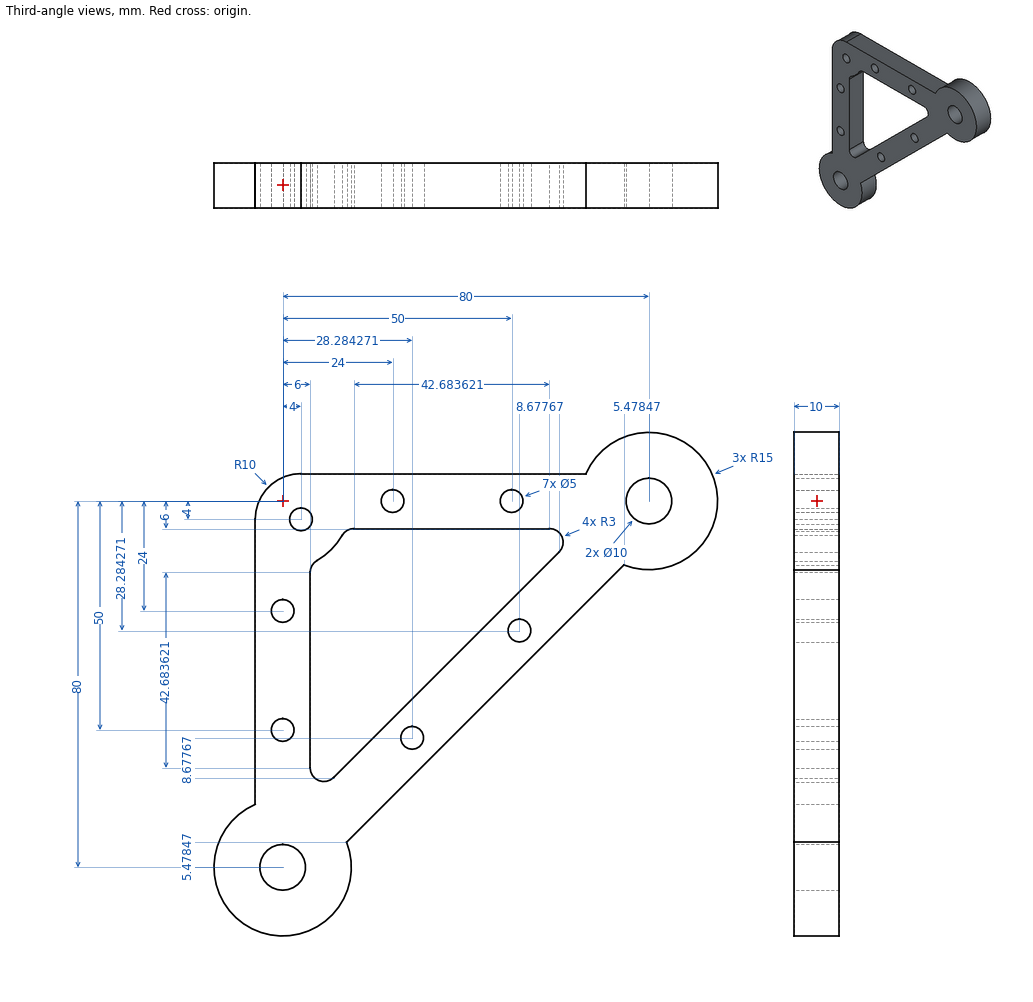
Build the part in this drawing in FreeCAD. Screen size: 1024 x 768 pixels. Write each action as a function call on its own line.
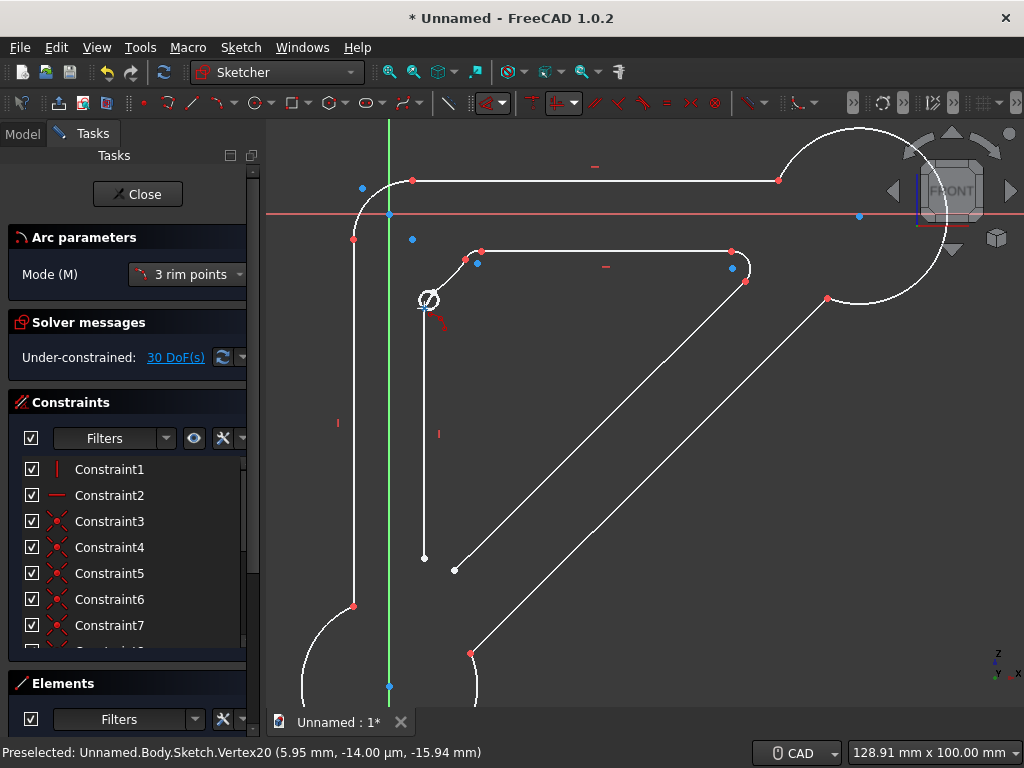
scroll(427, 297, up, 10)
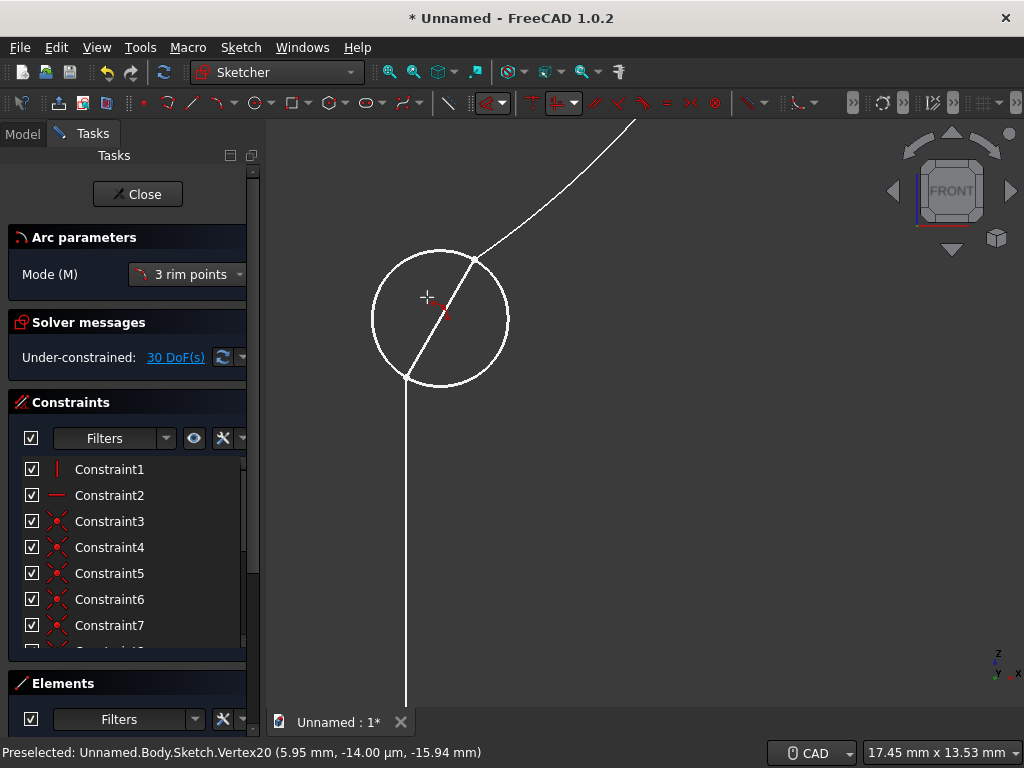
click(426, 297)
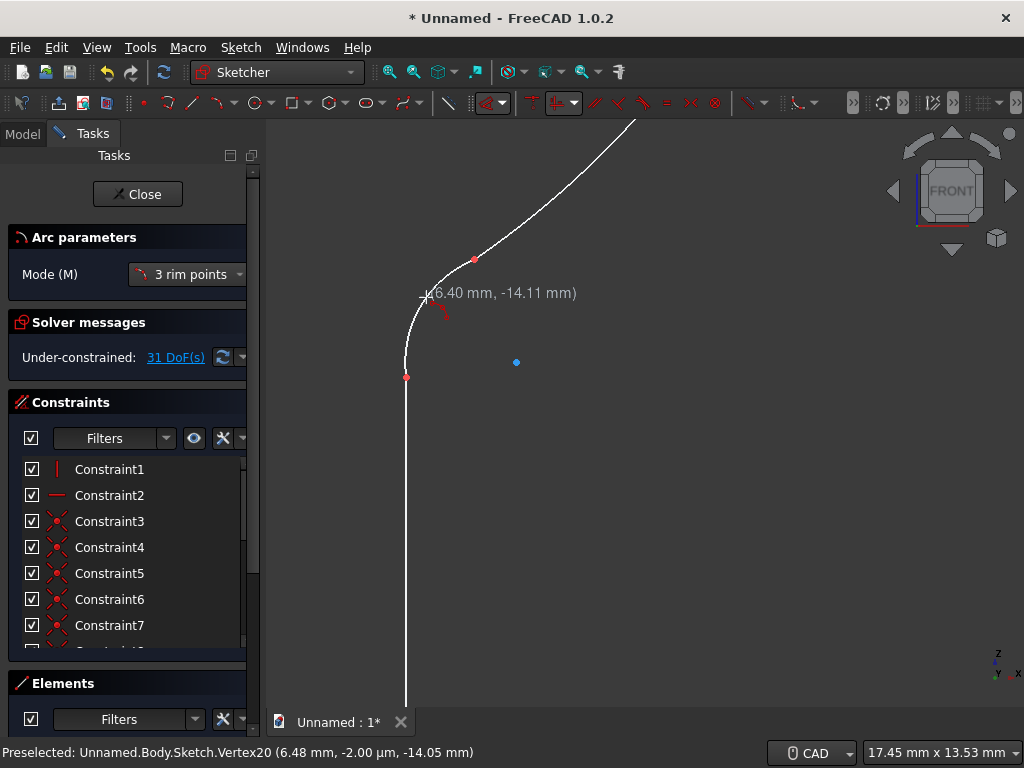
scroll(429, 295, down, 12)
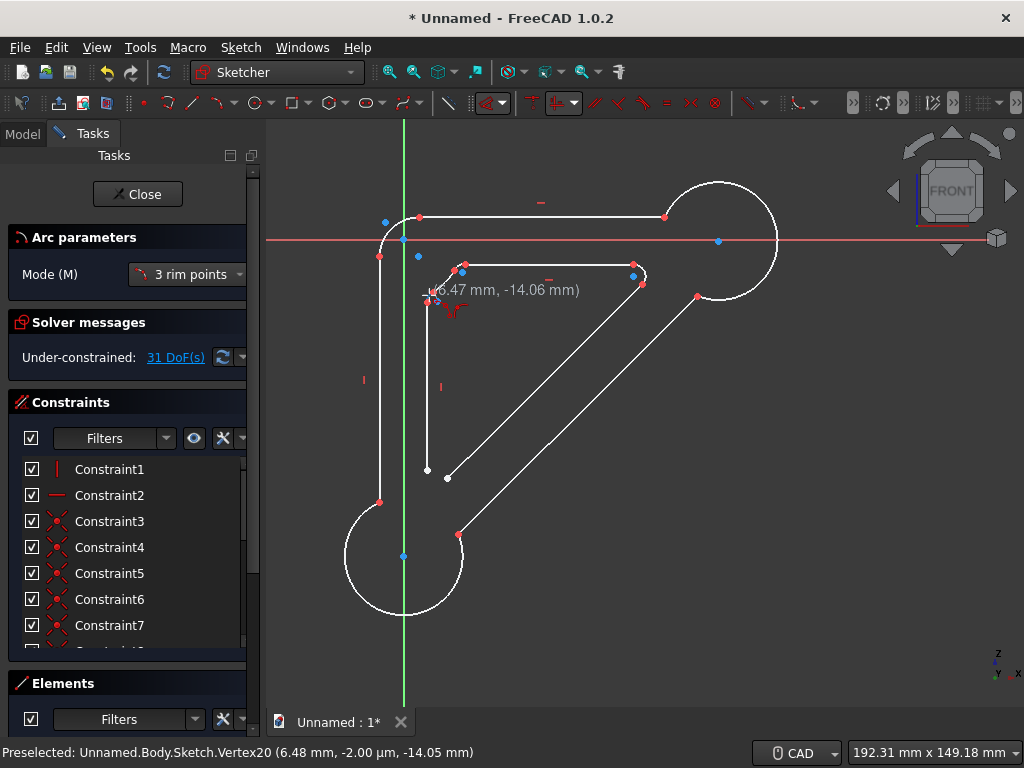
click(427, 471)
click(447, 479)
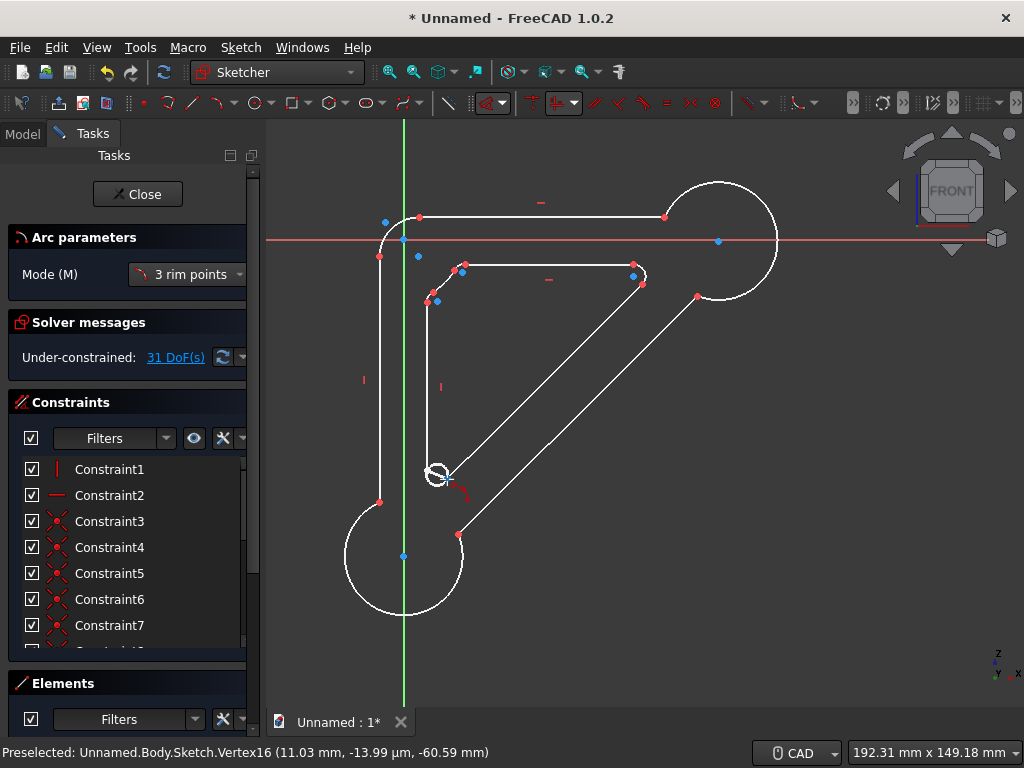
scroll(435, 481, up, 4)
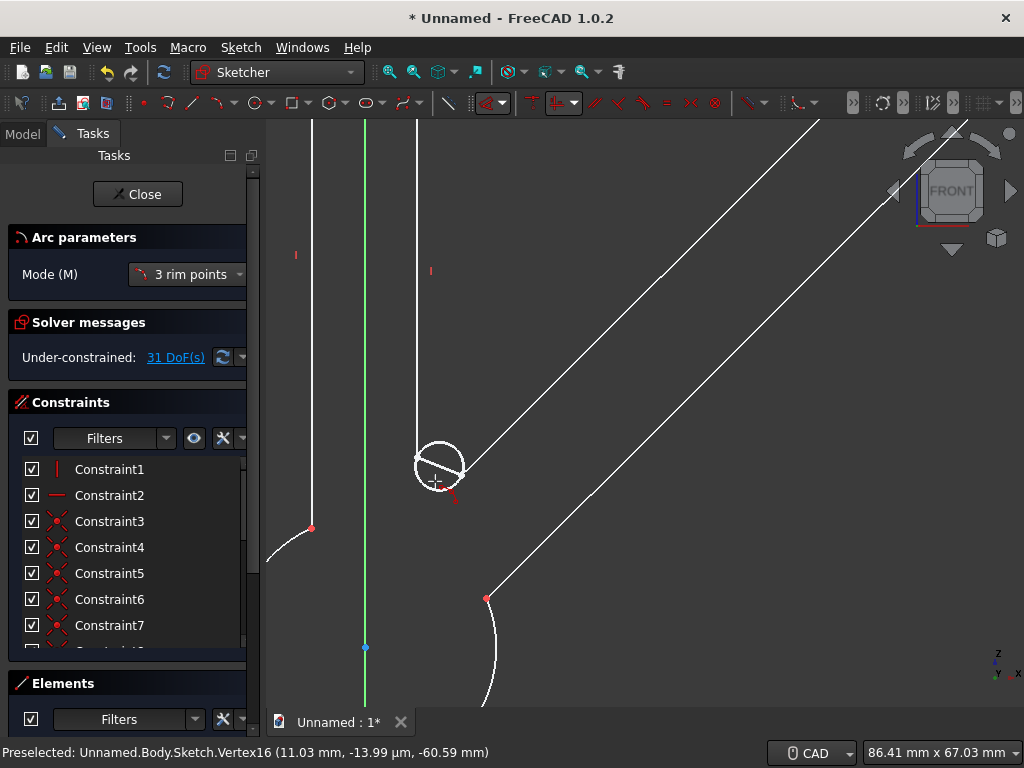
click(434, 479)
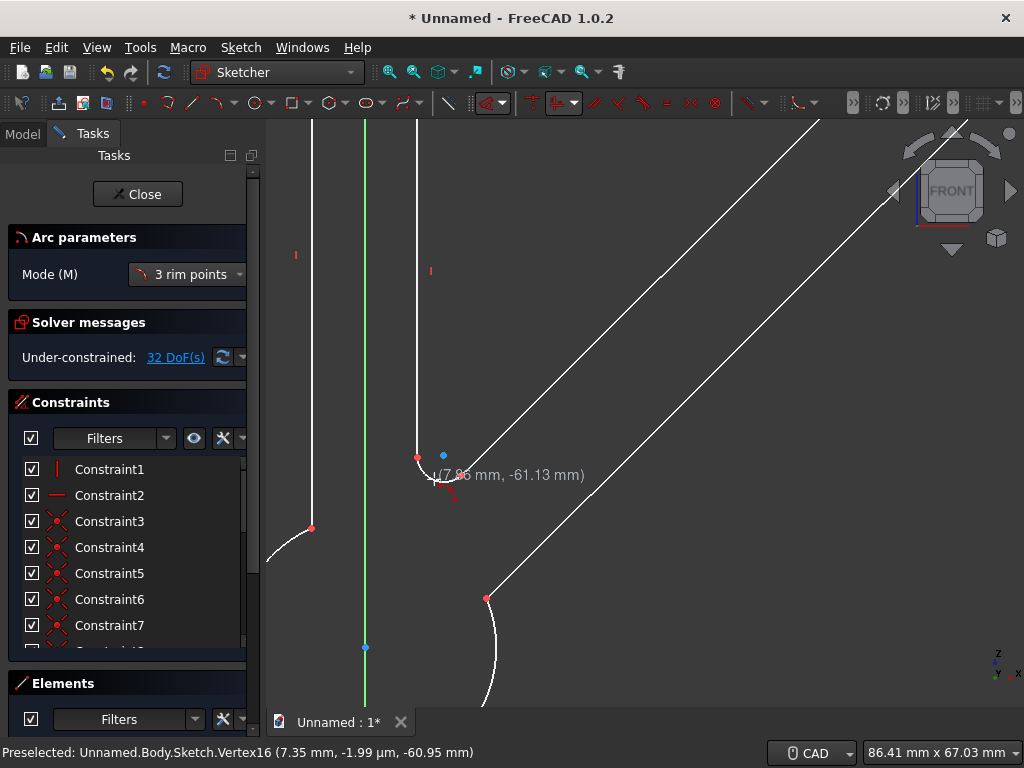
click(256, 104)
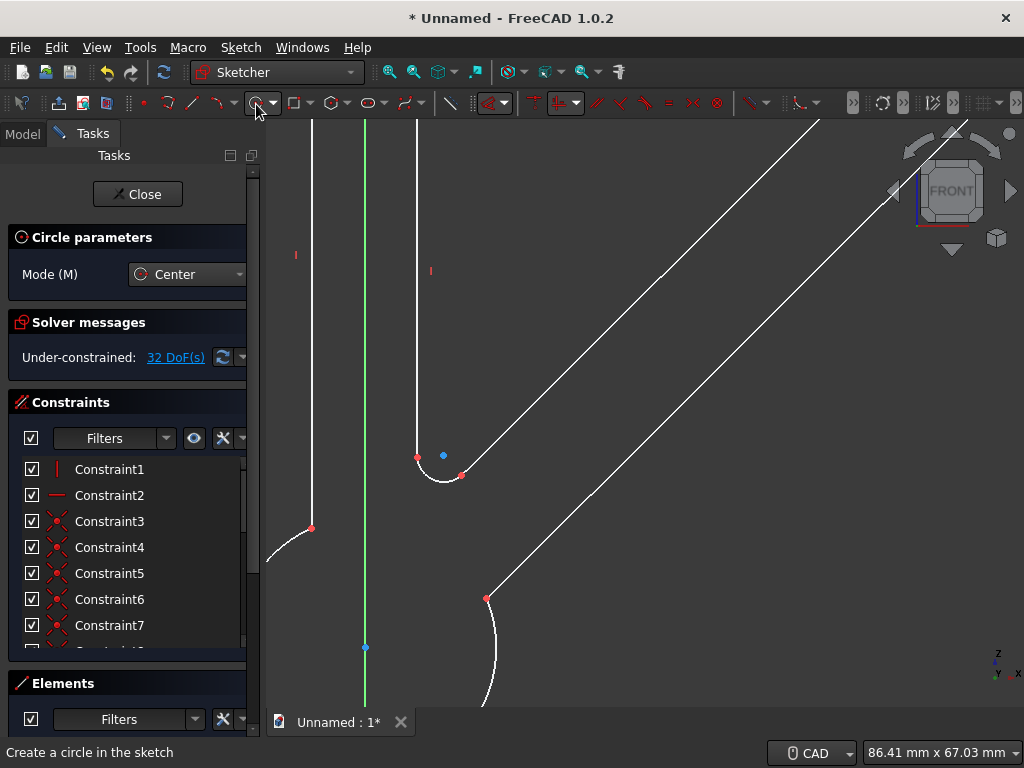
scroll(435, 481, down, 4)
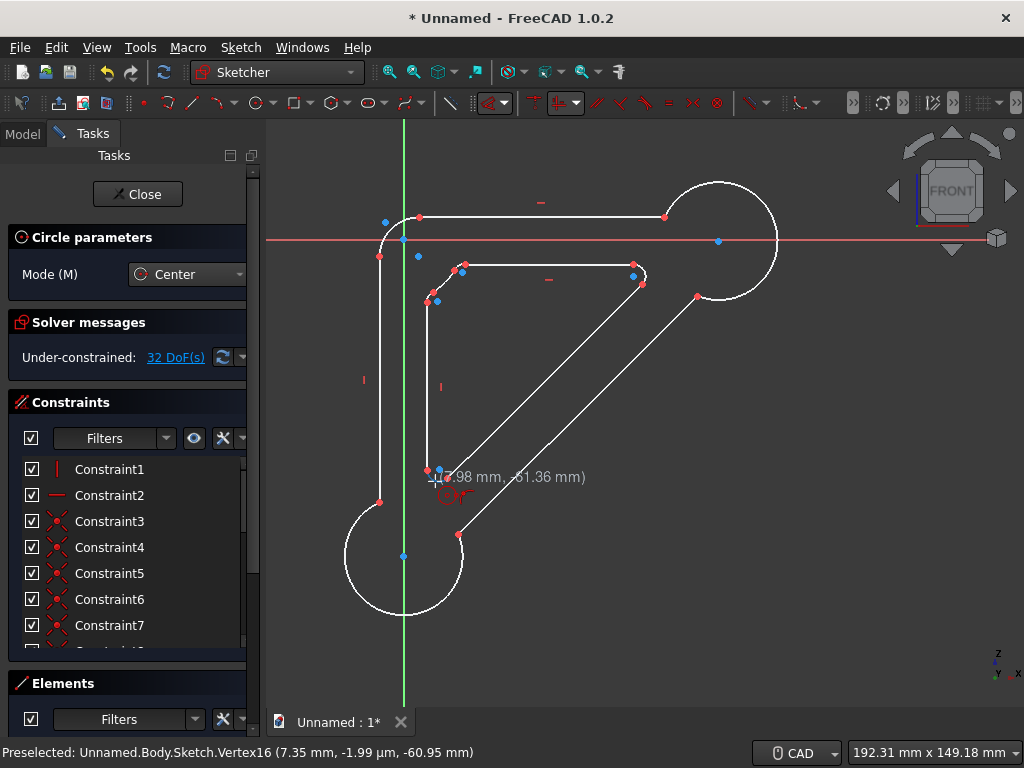
click(719, 240)
click(726, 221)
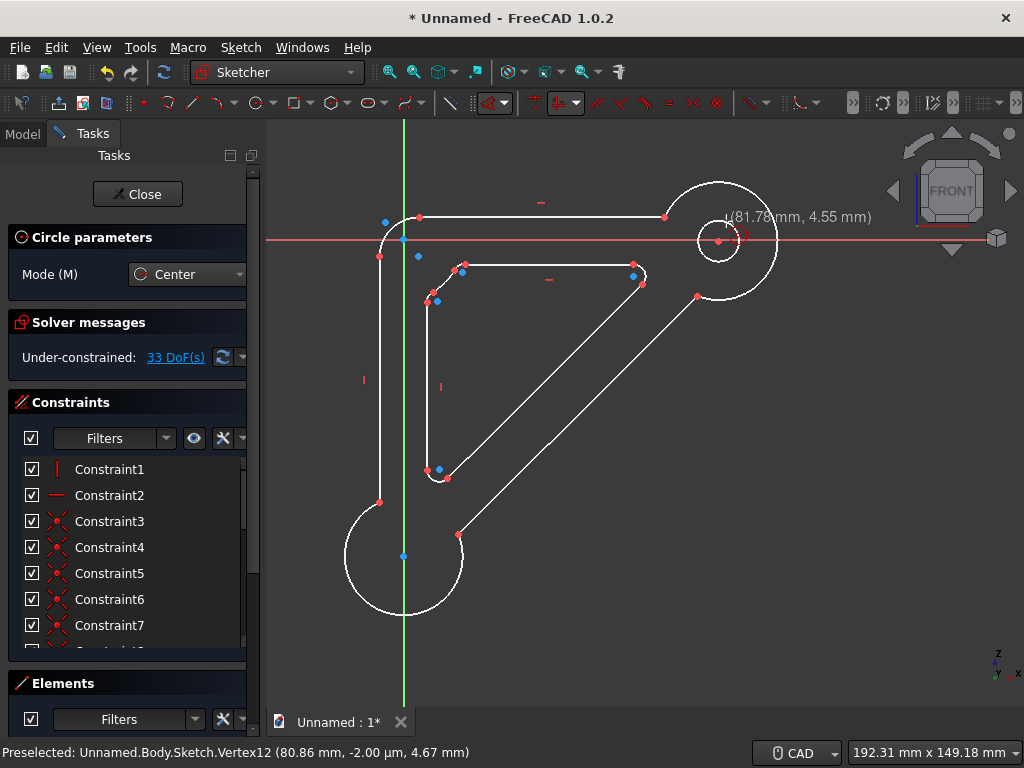
scroll(601, 240, up, 5)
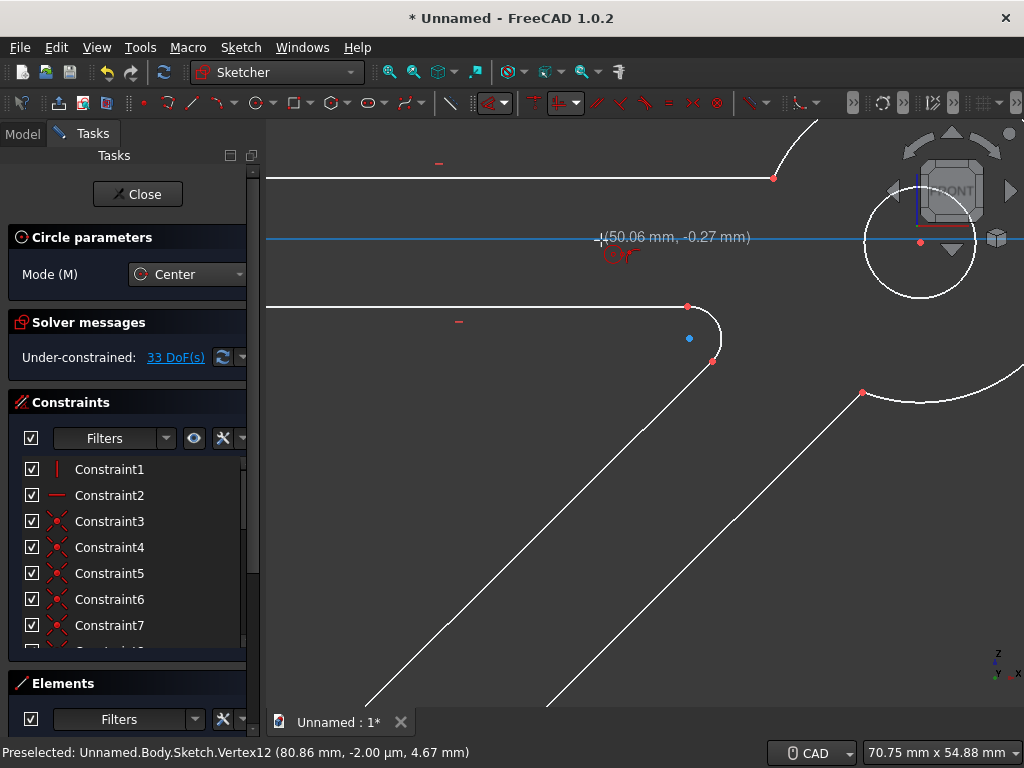
click(600, 239)
click(619, 221)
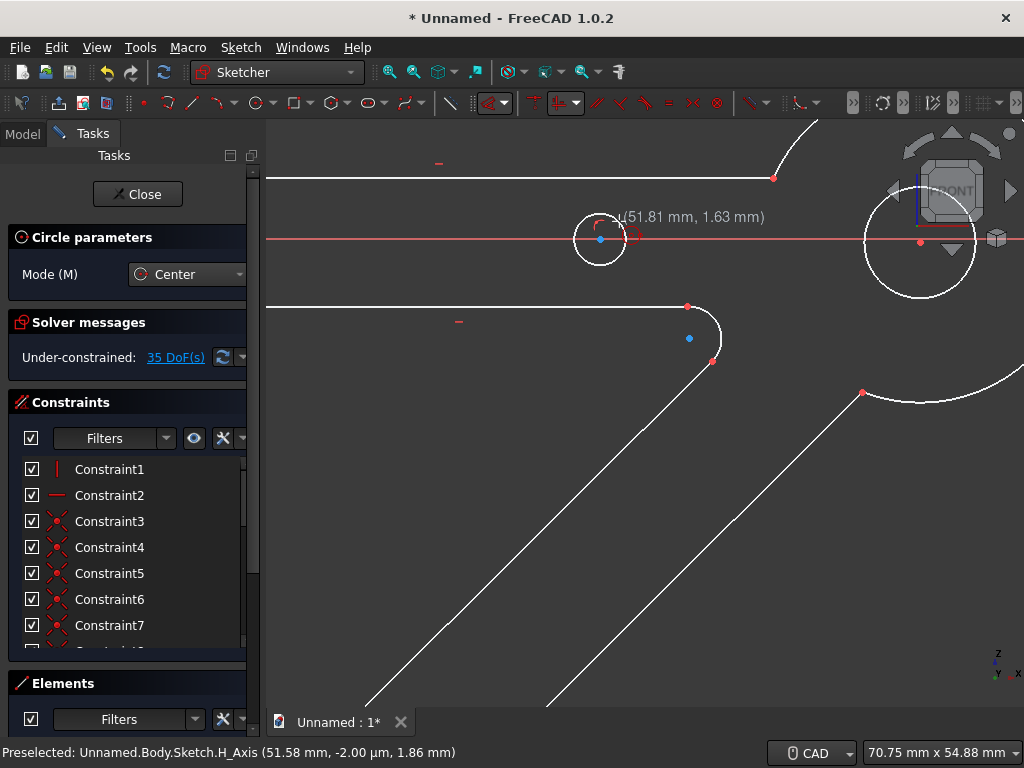
click(618, 543)
click(637, 524)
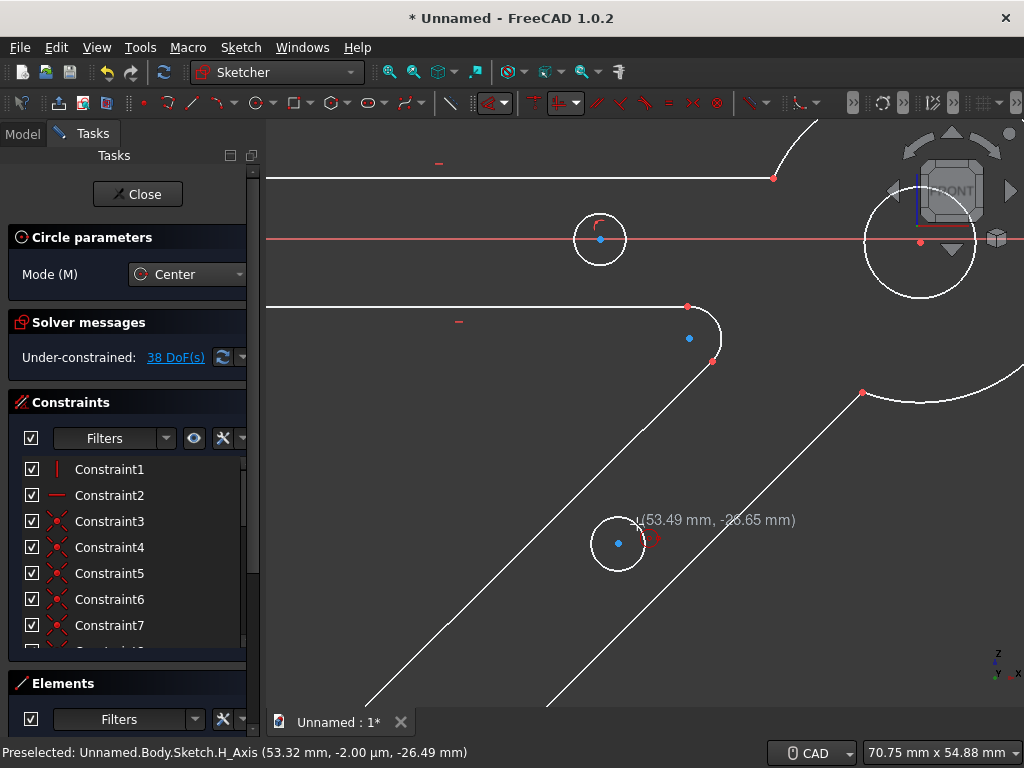
click(321, 239)
click(340, 221)